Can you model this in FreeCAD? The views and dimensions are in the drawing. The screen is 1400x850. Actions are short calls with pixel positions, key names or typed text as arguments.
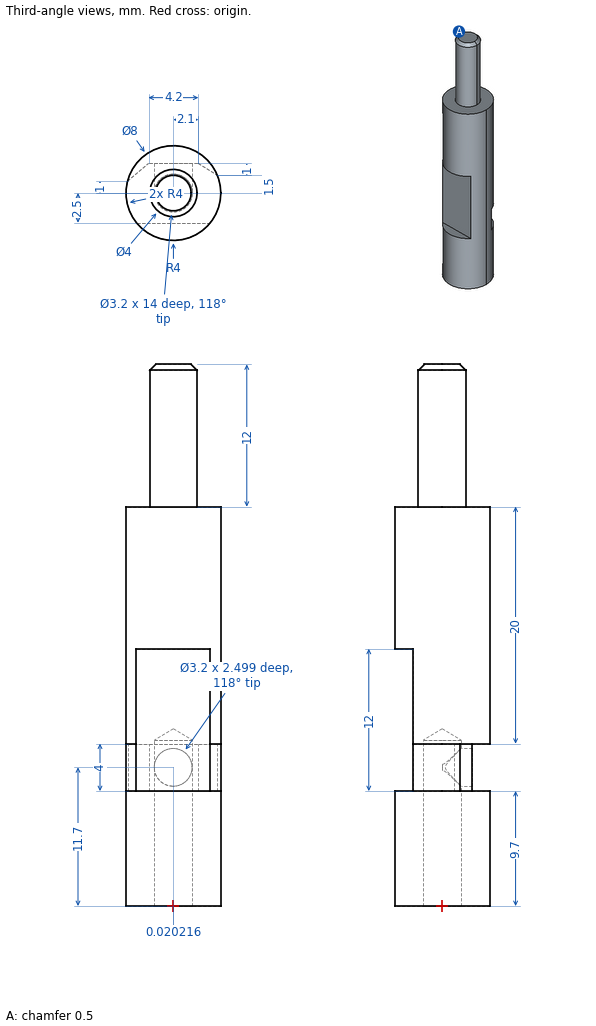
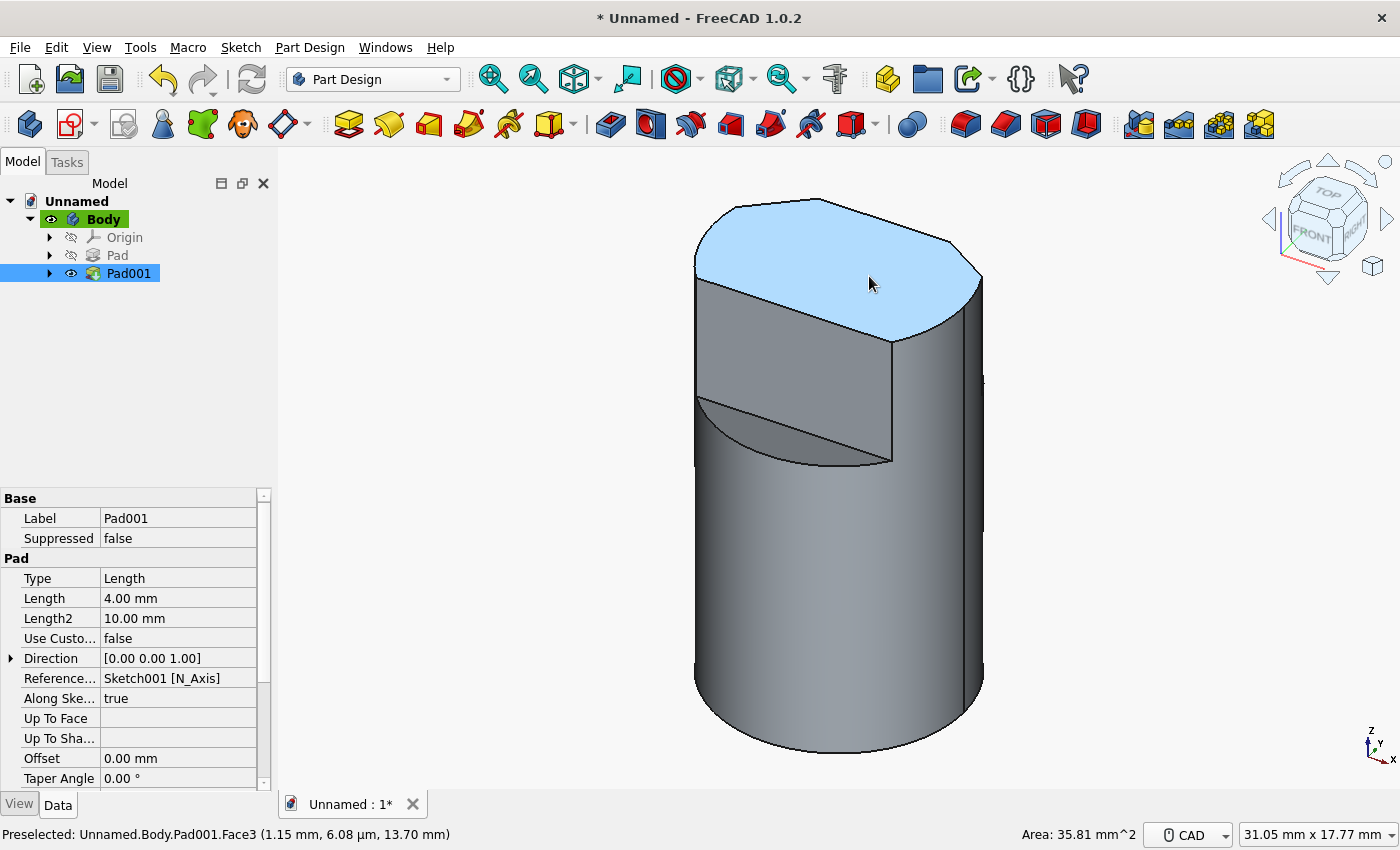
click(70, 124)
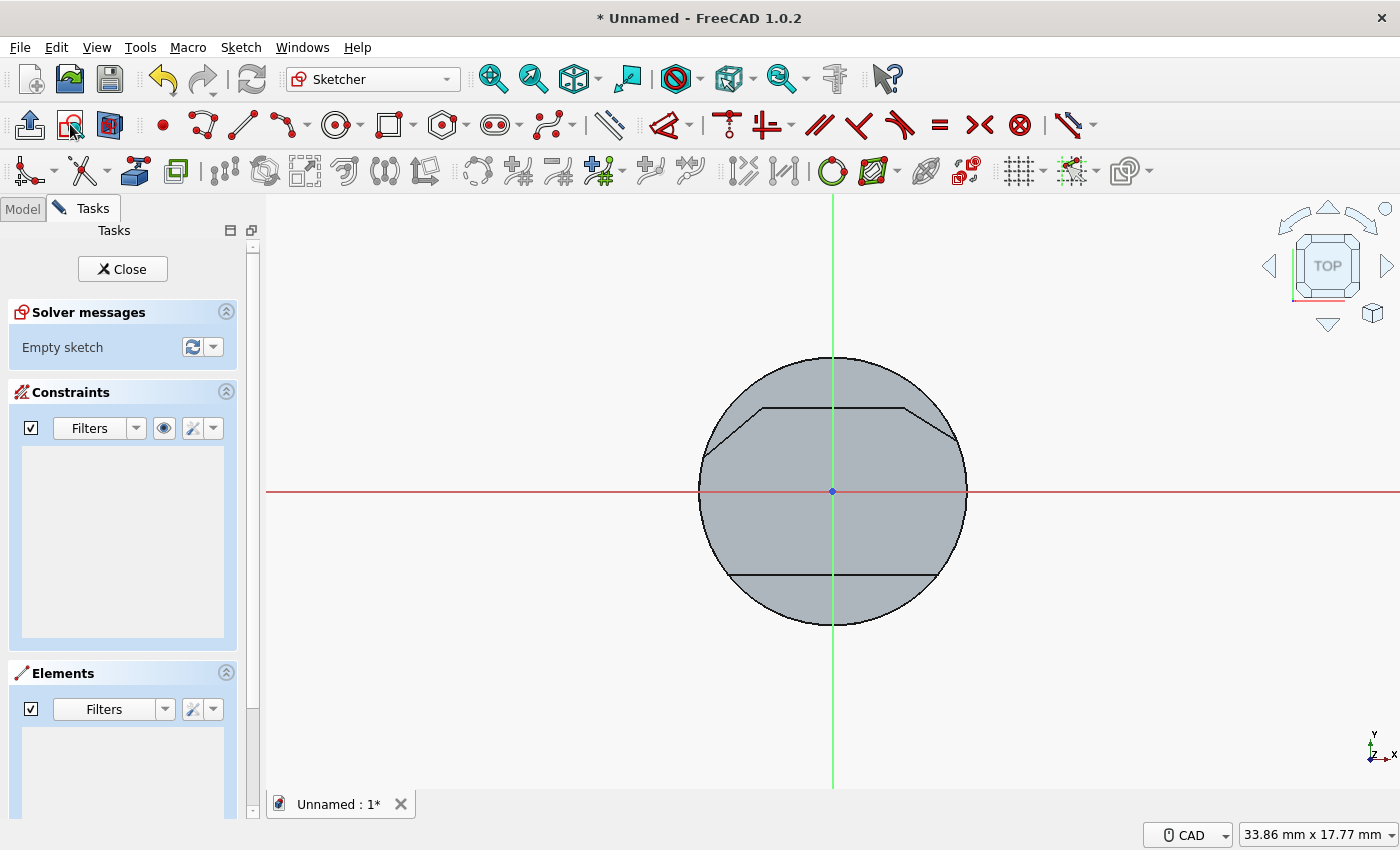
scroll(972, 491, up, 2)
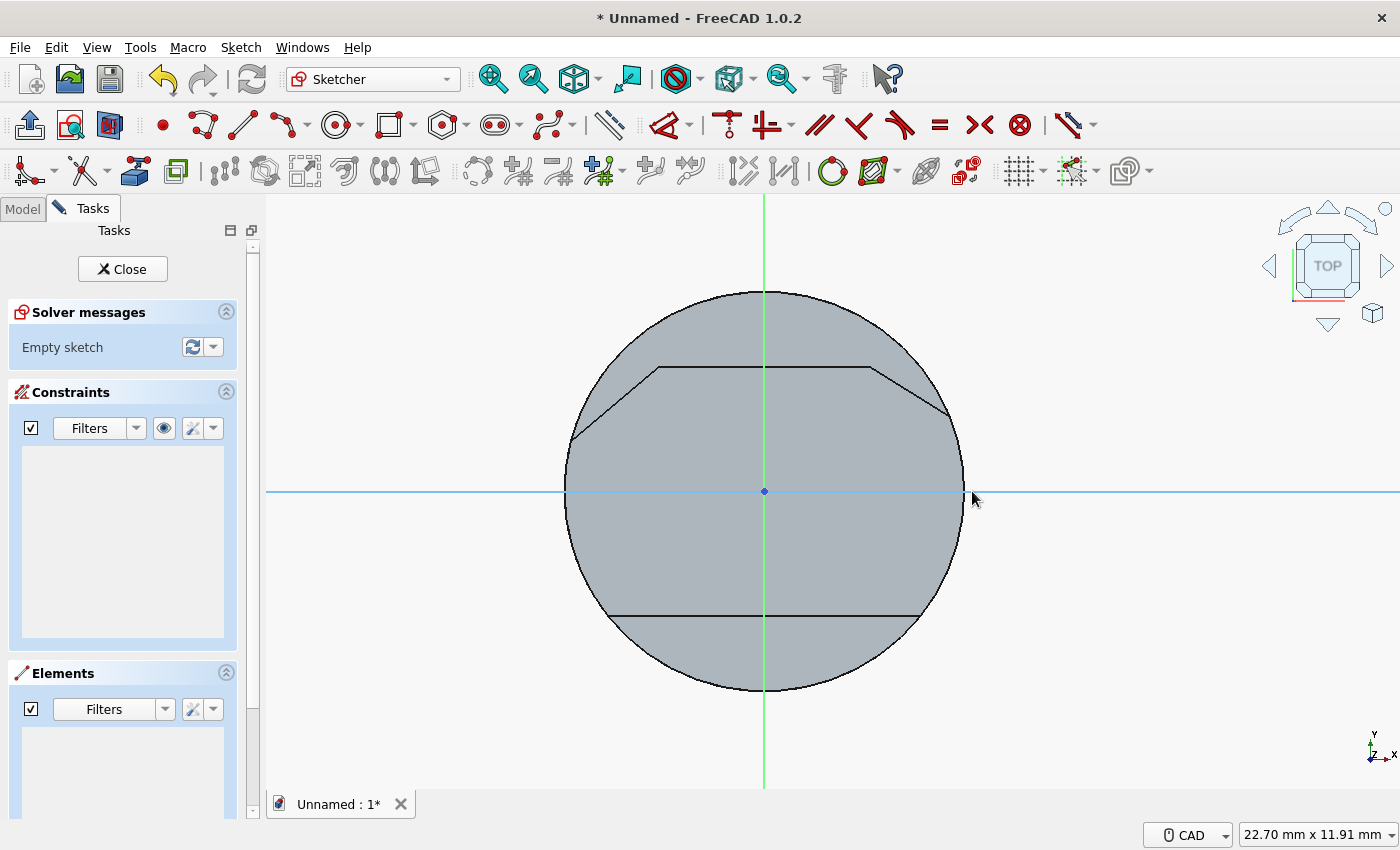
key(g)
key(c)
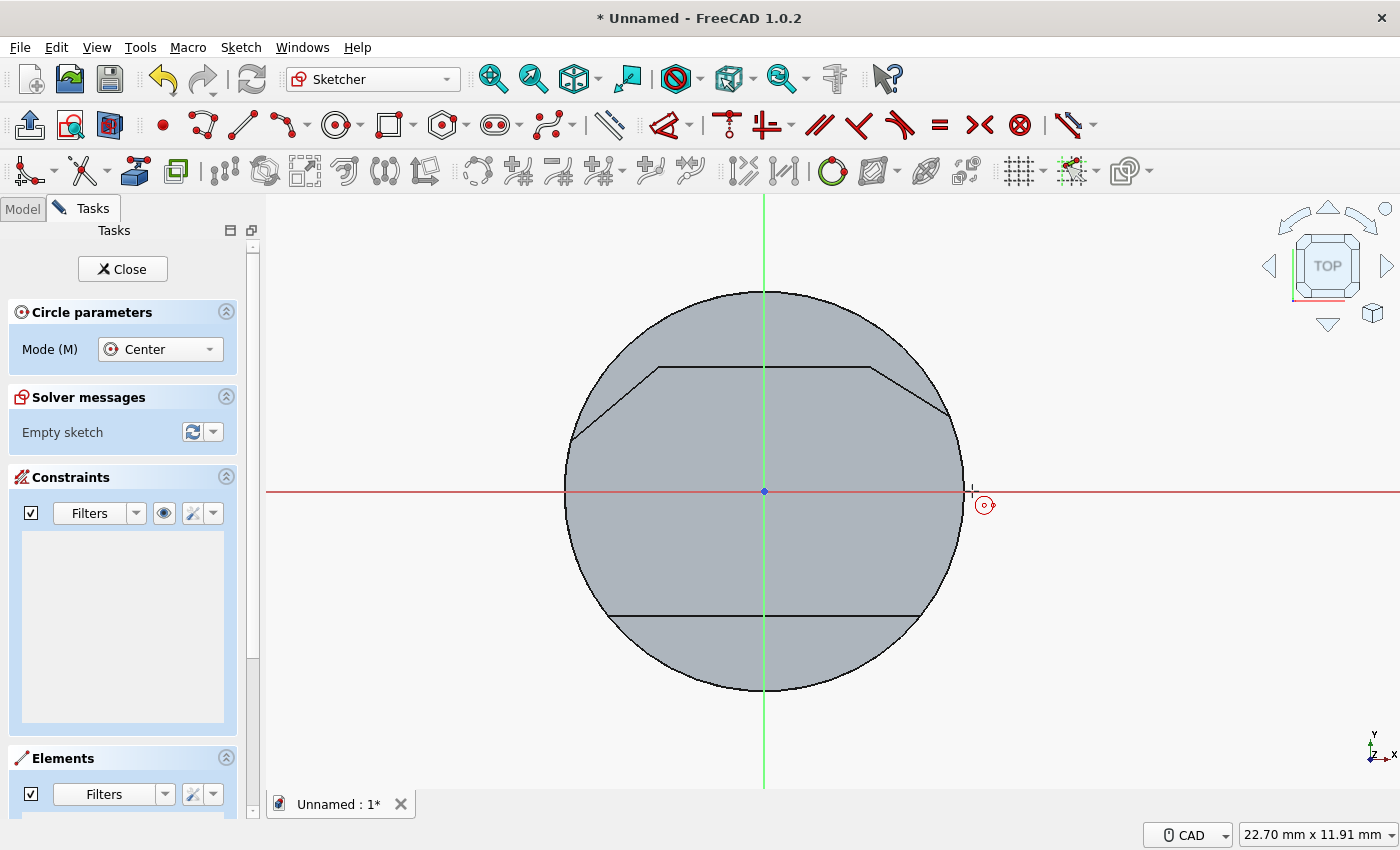
click(764, 492)
click(906, 350)
key(Escape)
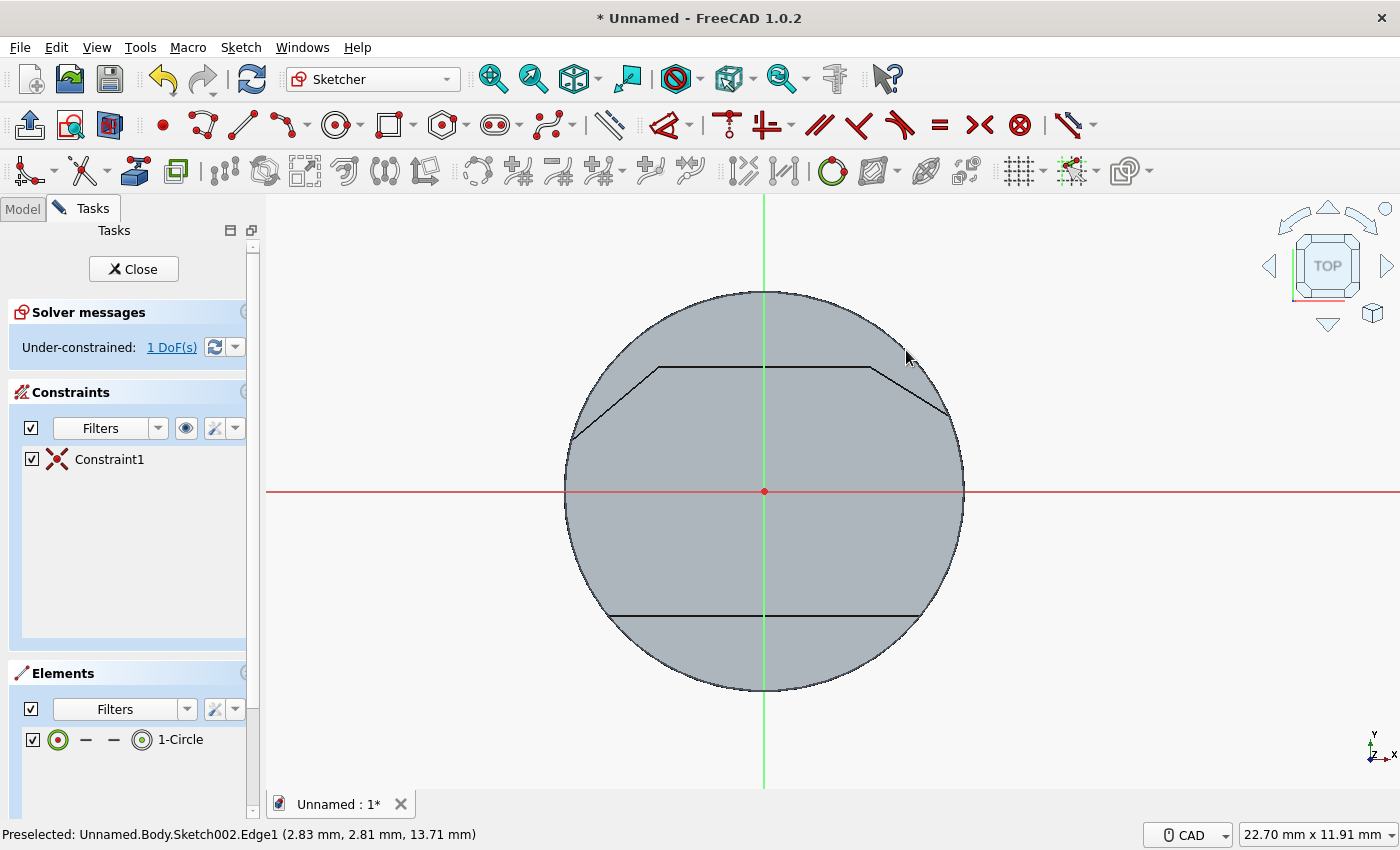
click(664, 126)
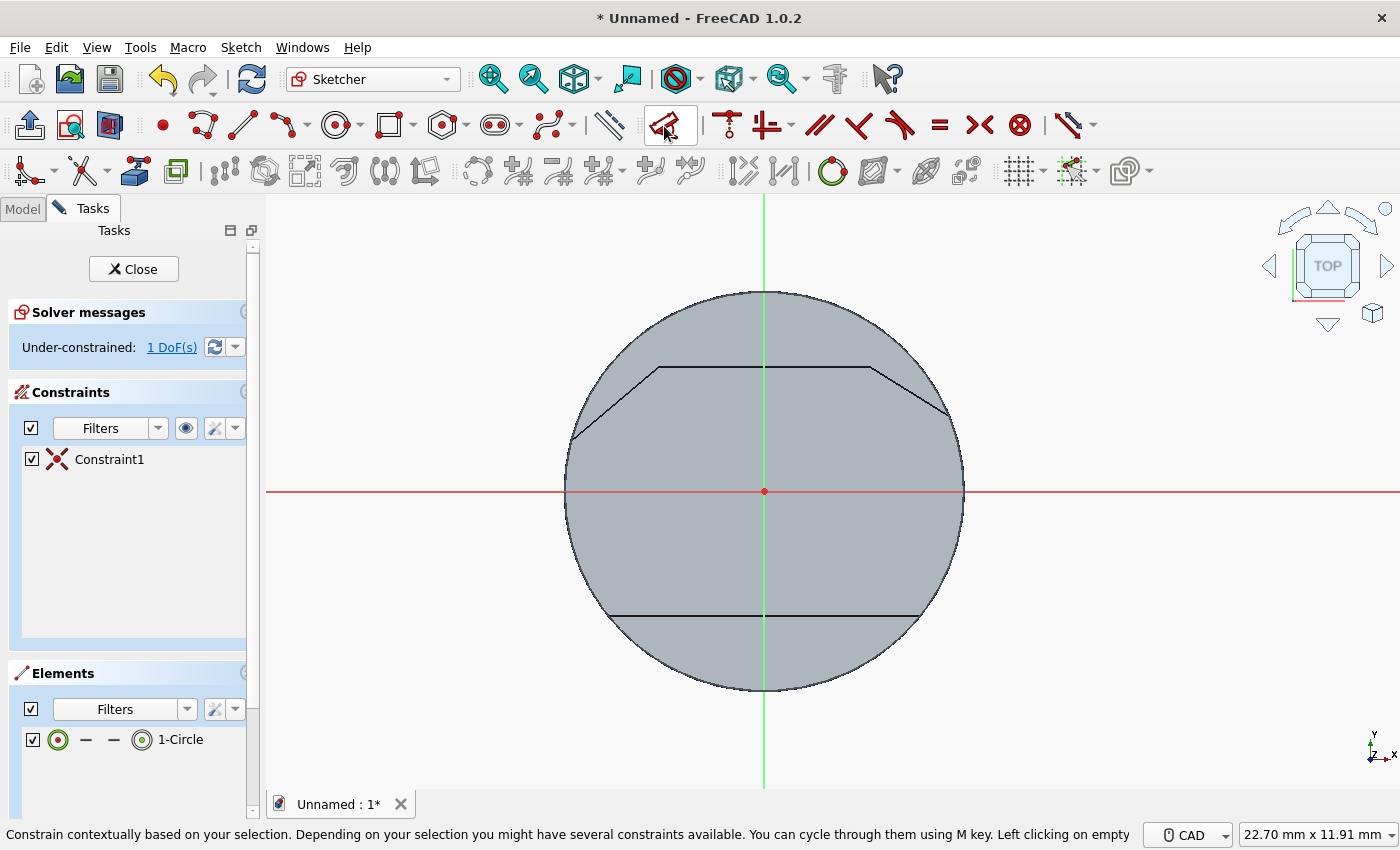
click(905, 350)
click(928, 327)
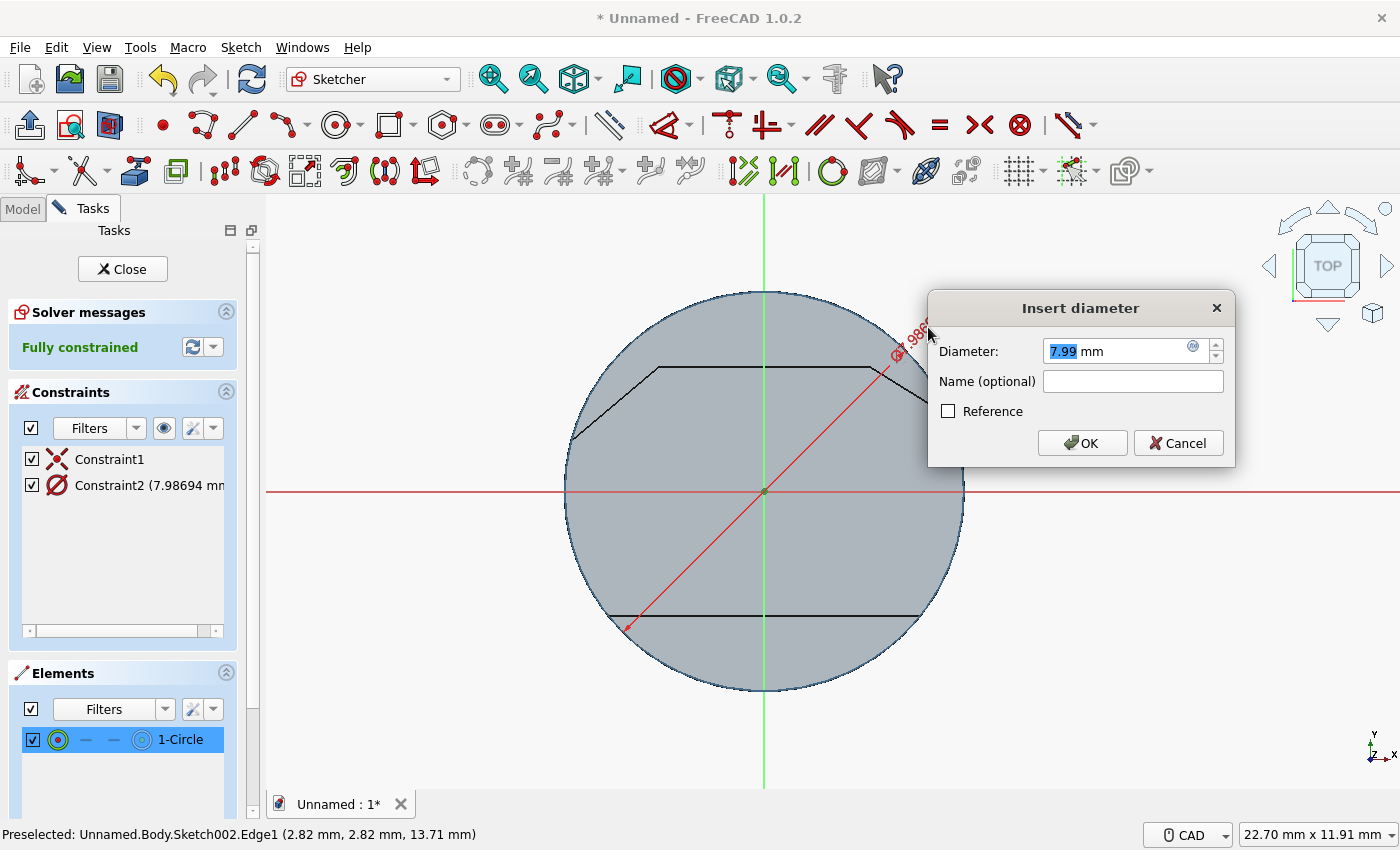
text(8)
key(Return)
key(Escape)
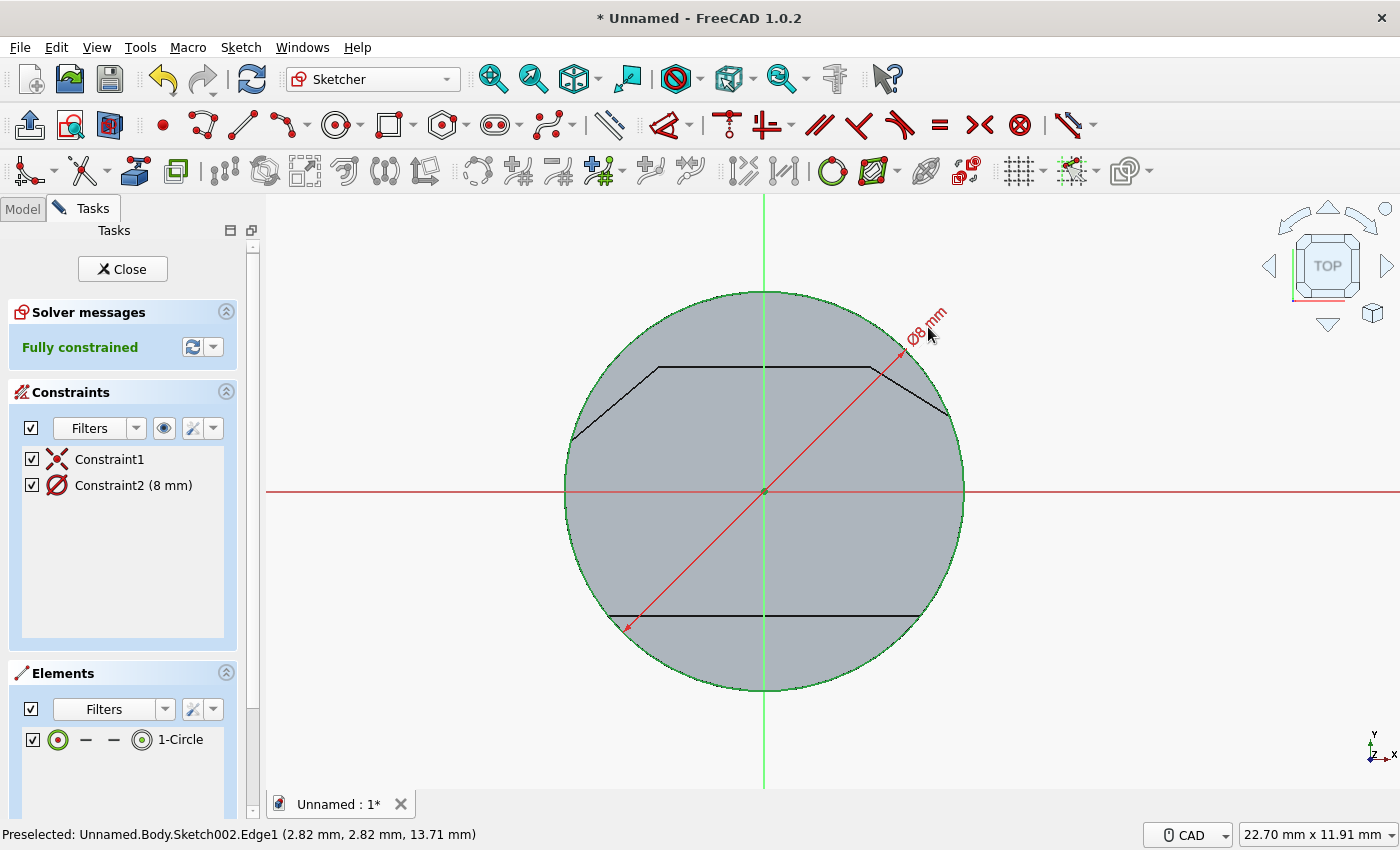
click(123, 269)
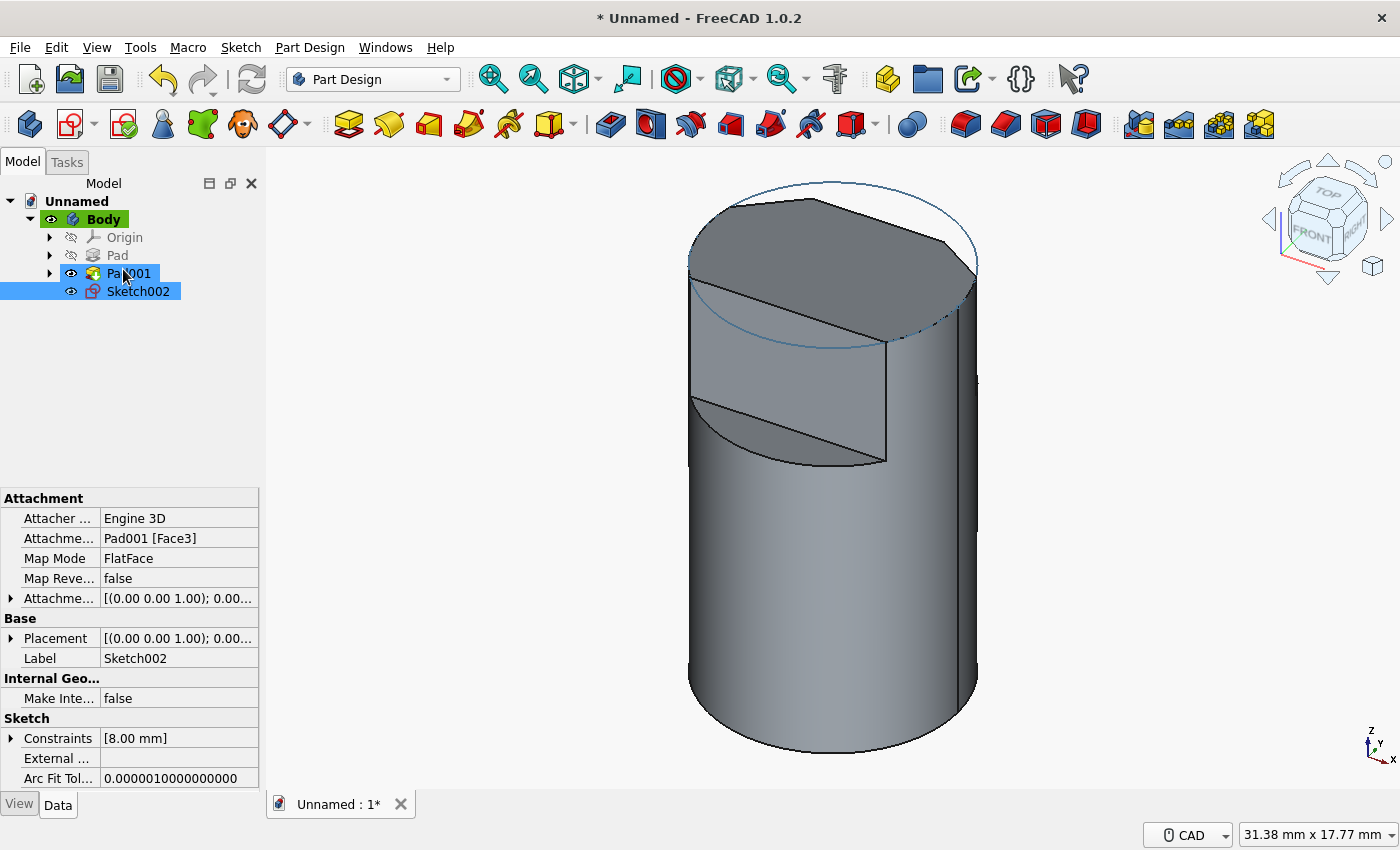
click(350, 124)